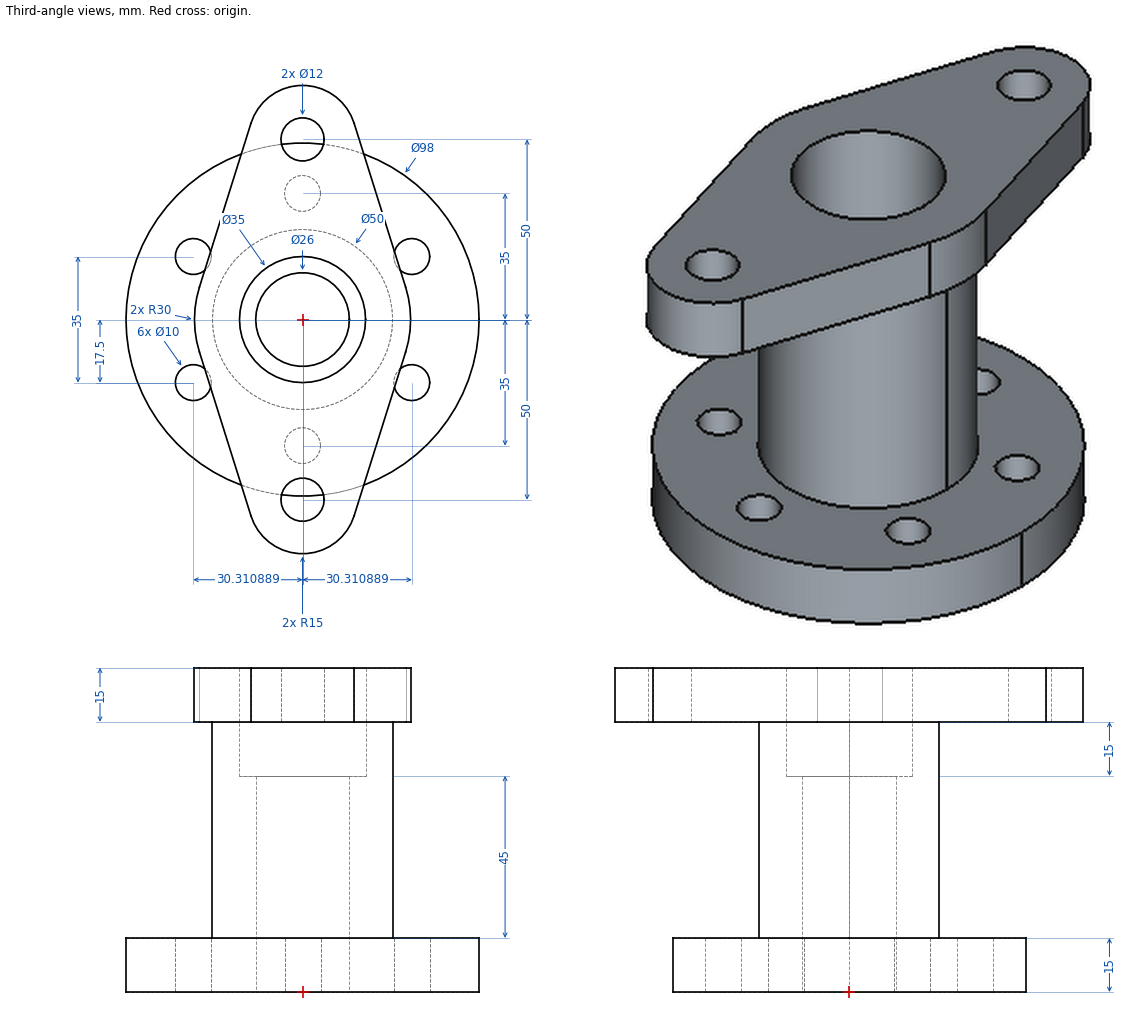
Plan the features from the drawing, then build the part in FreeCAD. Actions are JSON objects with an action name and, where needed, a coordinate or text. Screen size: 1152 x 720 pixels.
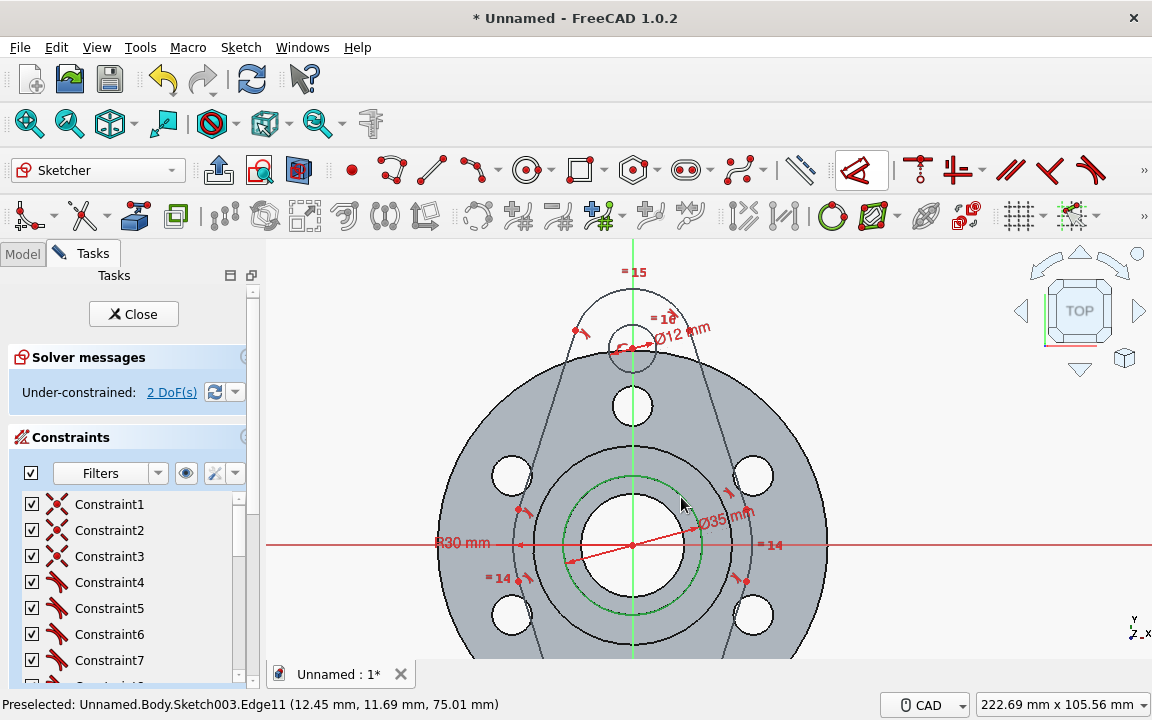
{"action": "left_click", "coordinate": [633, 349]}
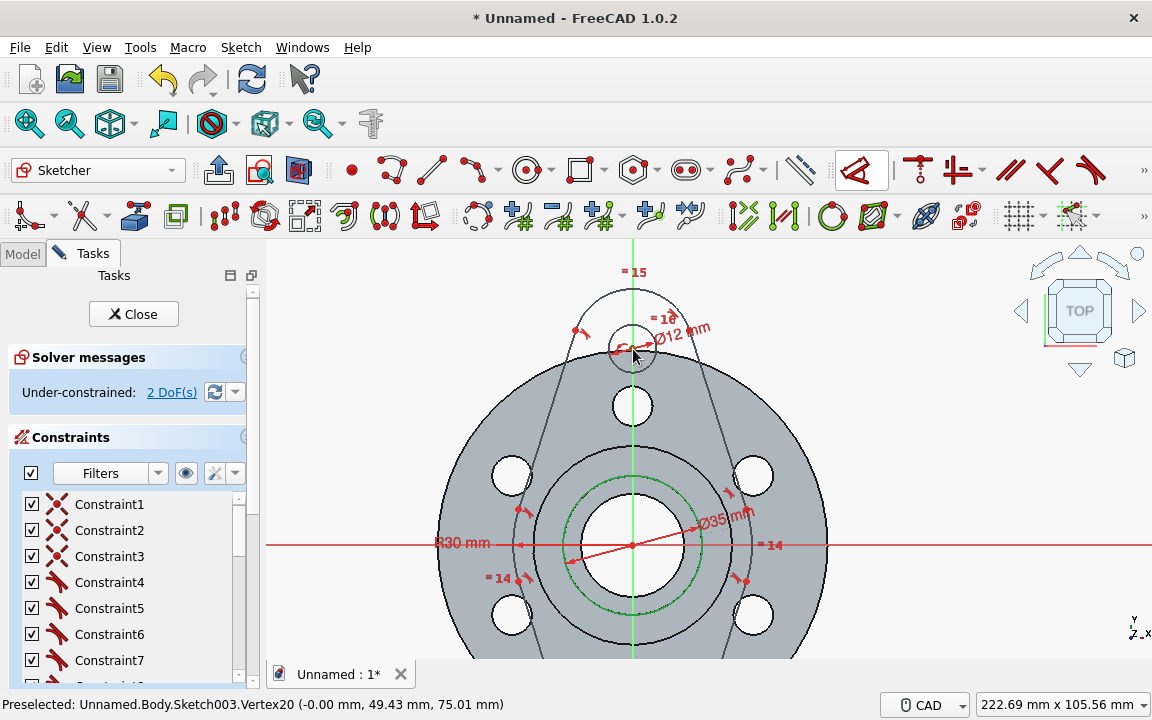
{"action": "key", "text": "i"}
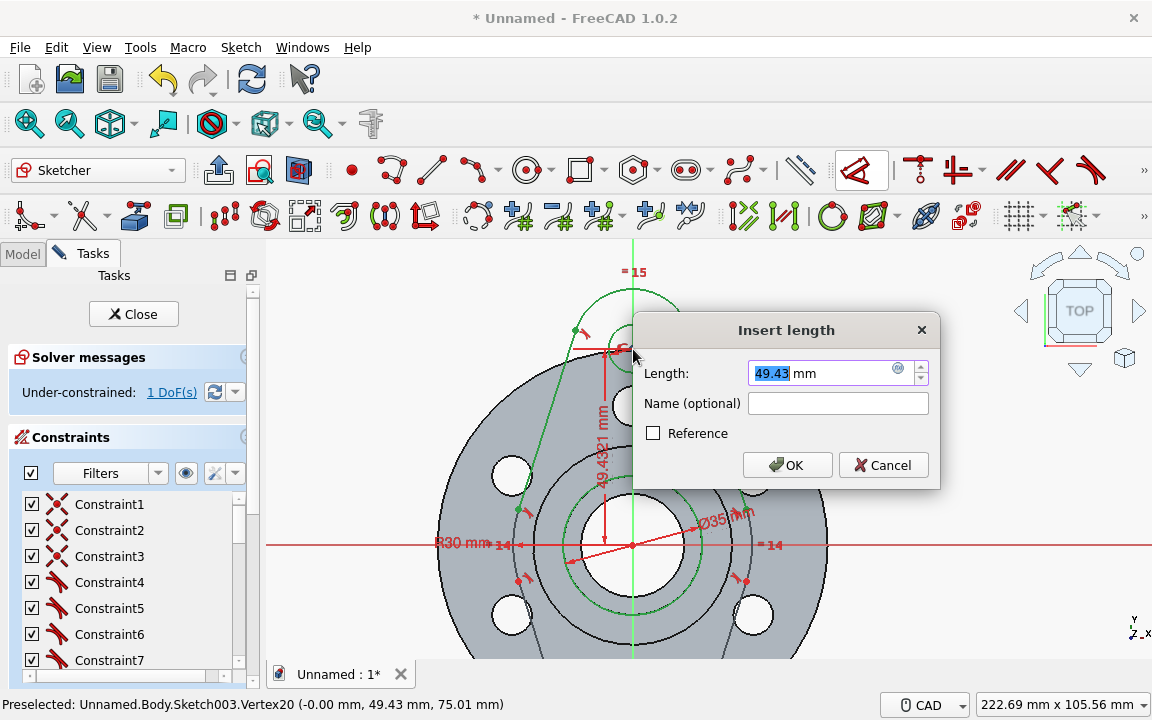
{"action": "type", "text": "50"}
{"action": "key", "text": "Return"}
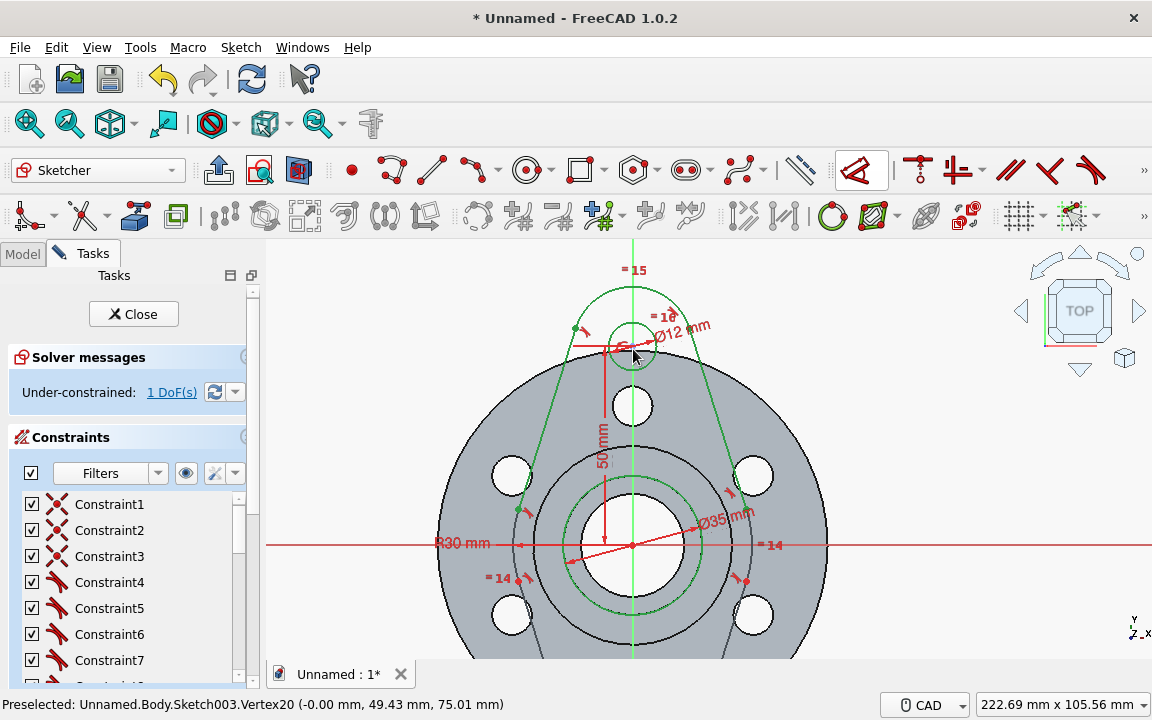
{"action": "scroll", "coordinate": [650, 332], "scroll_direction": "down", "scroll_amount": 3}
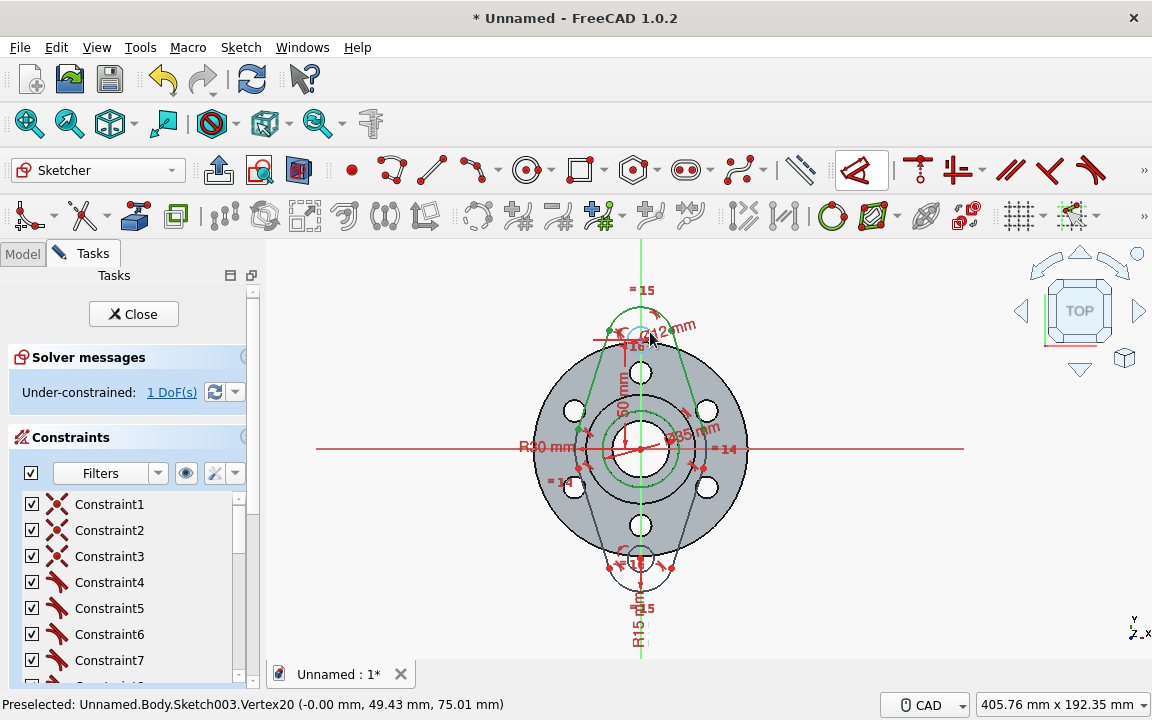
{"action": "left_click", "coordinate": [641, 559]}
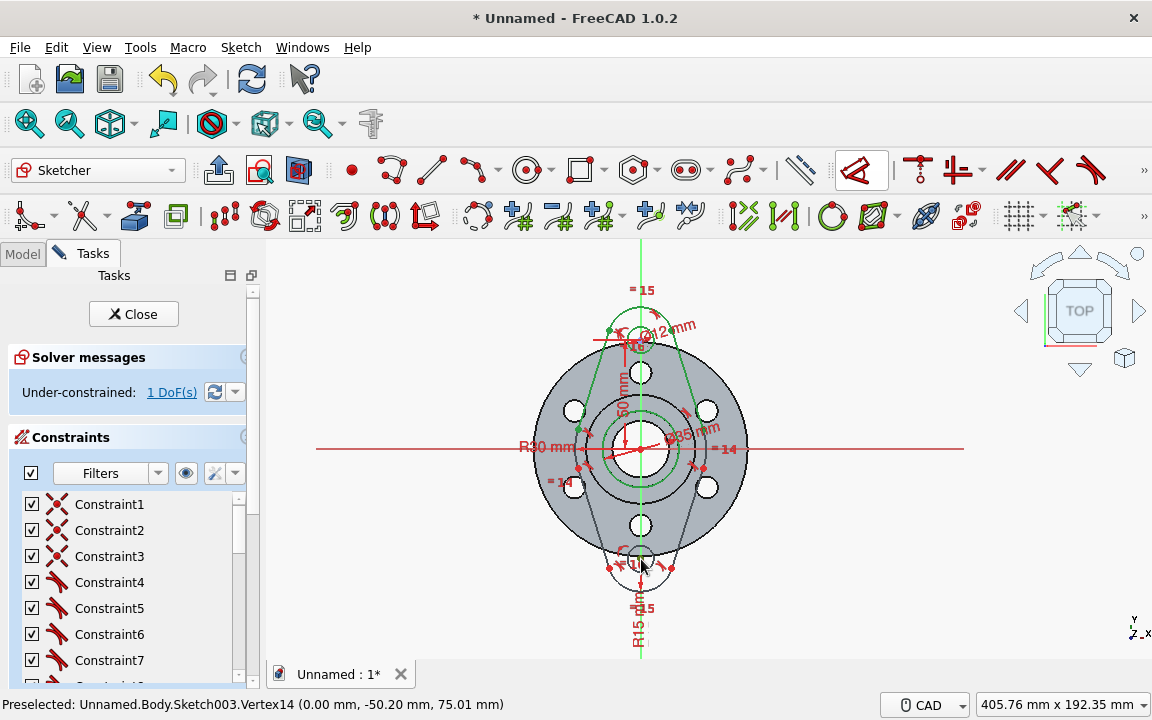
{"action": "key", "text": "i"}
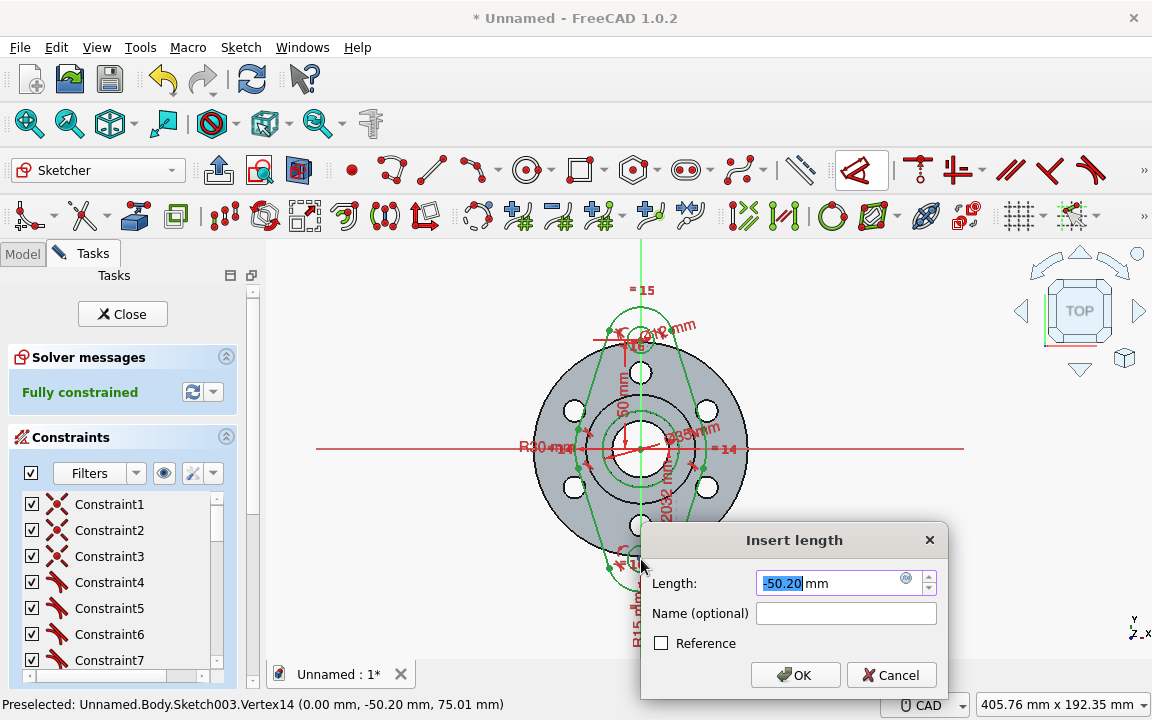
{"action": "type", "text": "-50"}
{"action": "key", "text": "Return"}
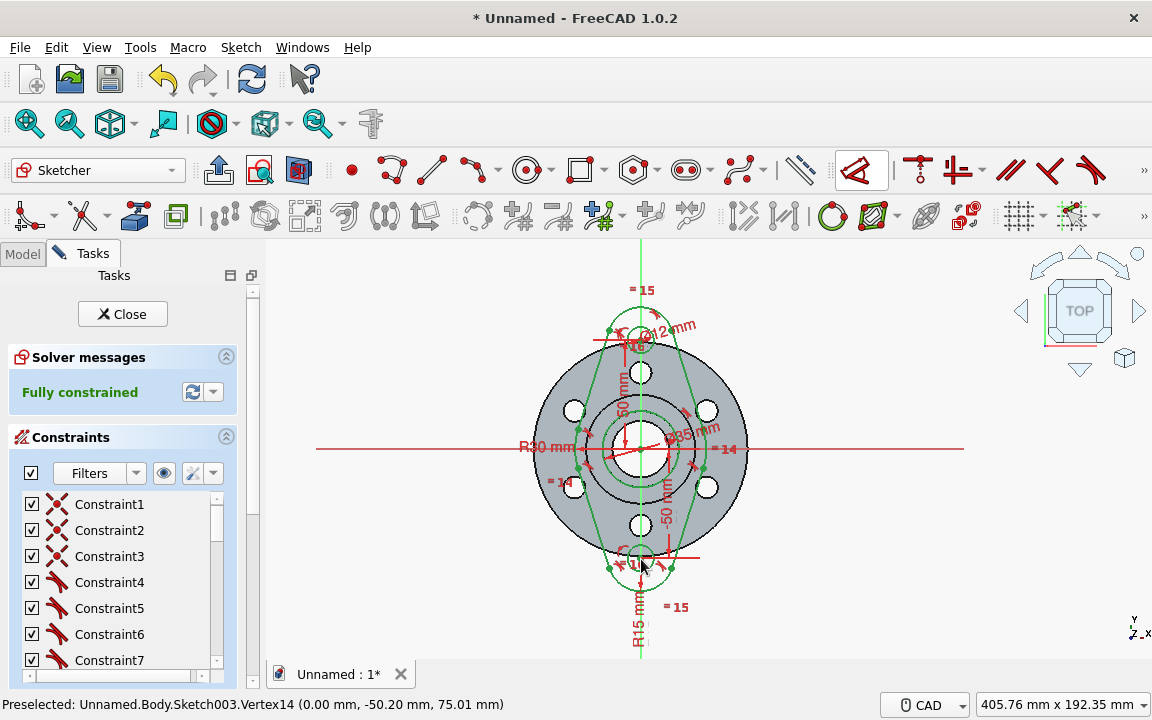
{"action": "left_click", "coordinate": [123, 314]}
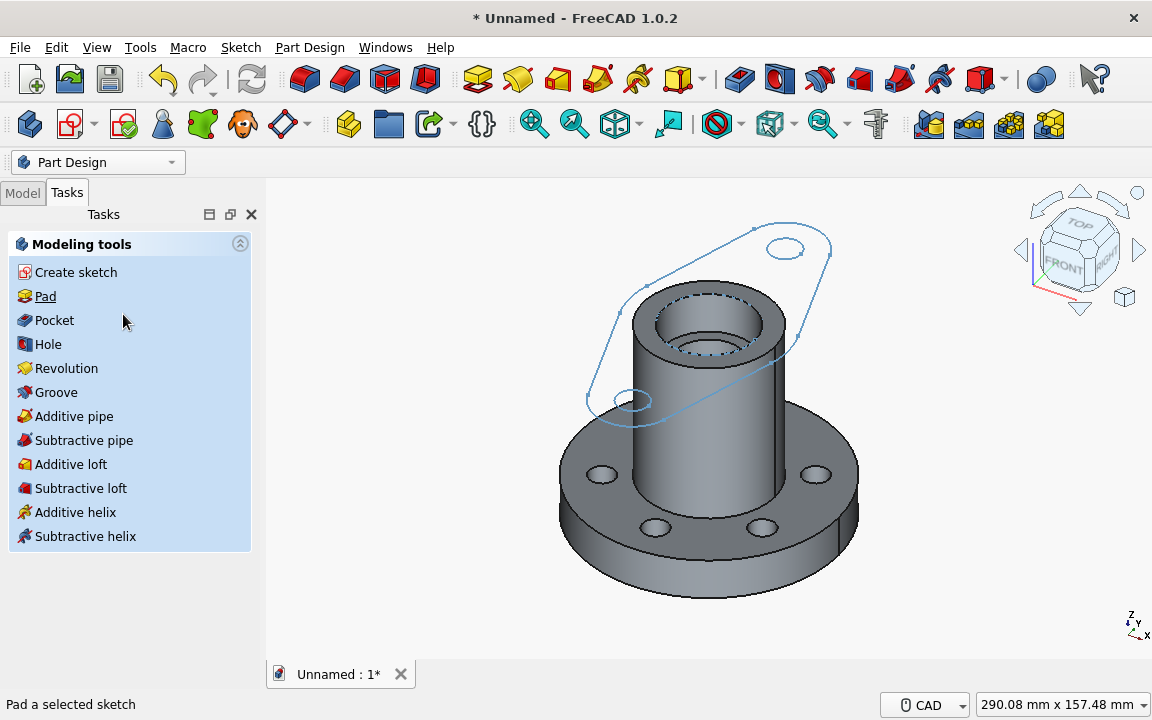
{"action": "left_click", "coordinate": [478, 80]}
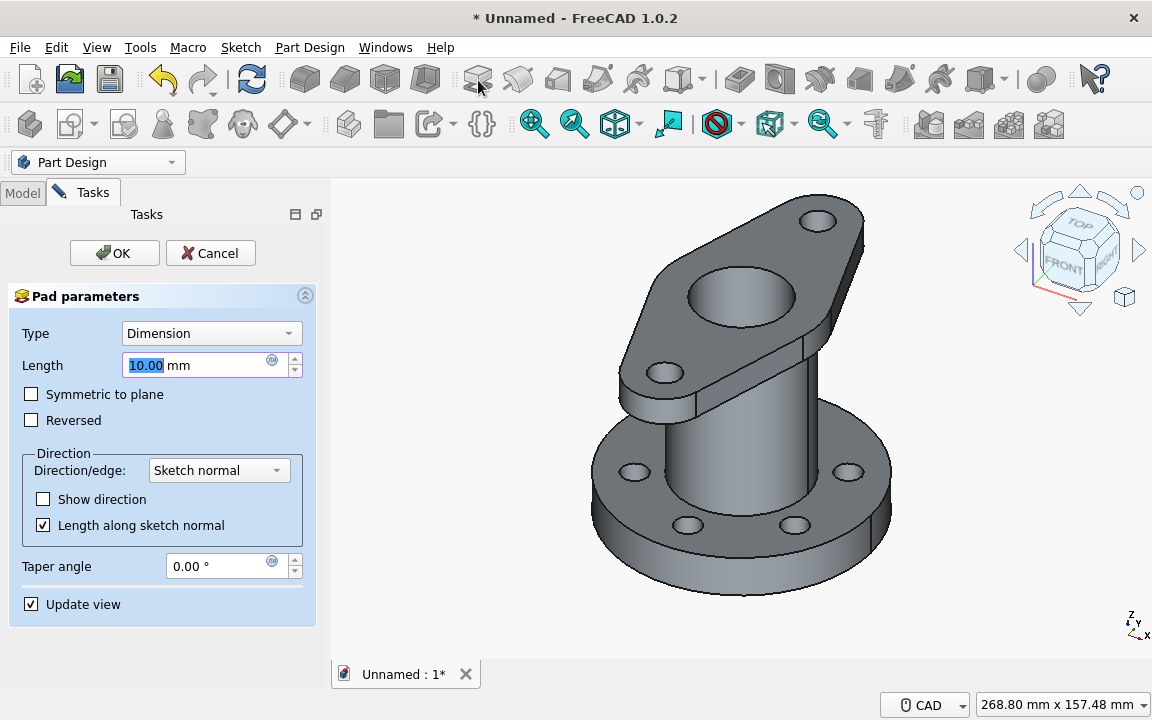
{"action": "type", "text": "15"}
{"action": "key", "text": "Tab"}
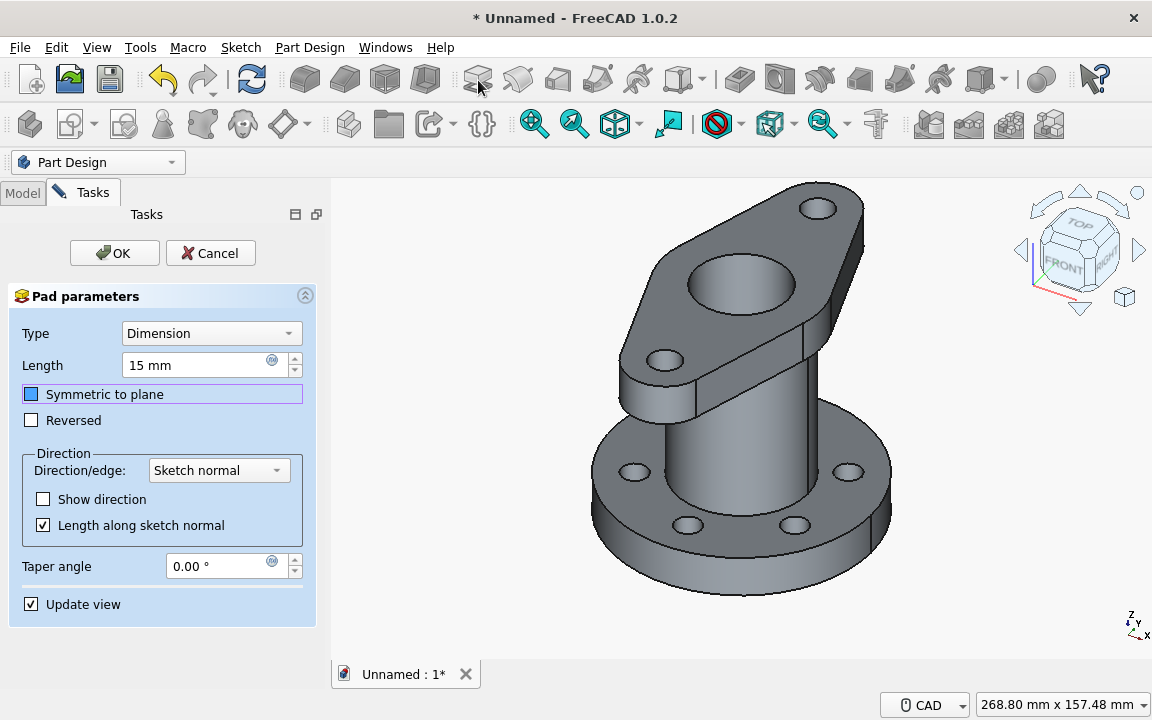
{"action": "left_click", "coordinate": [115, 253]}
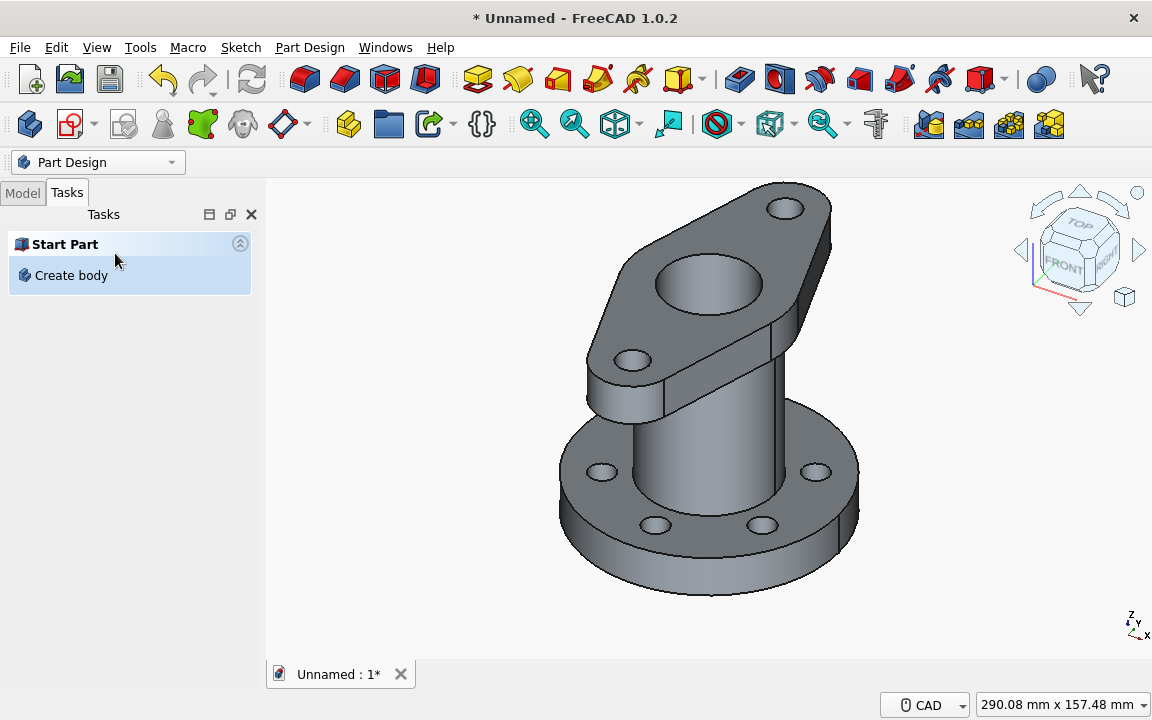
{"action": "key", "text": "0"}